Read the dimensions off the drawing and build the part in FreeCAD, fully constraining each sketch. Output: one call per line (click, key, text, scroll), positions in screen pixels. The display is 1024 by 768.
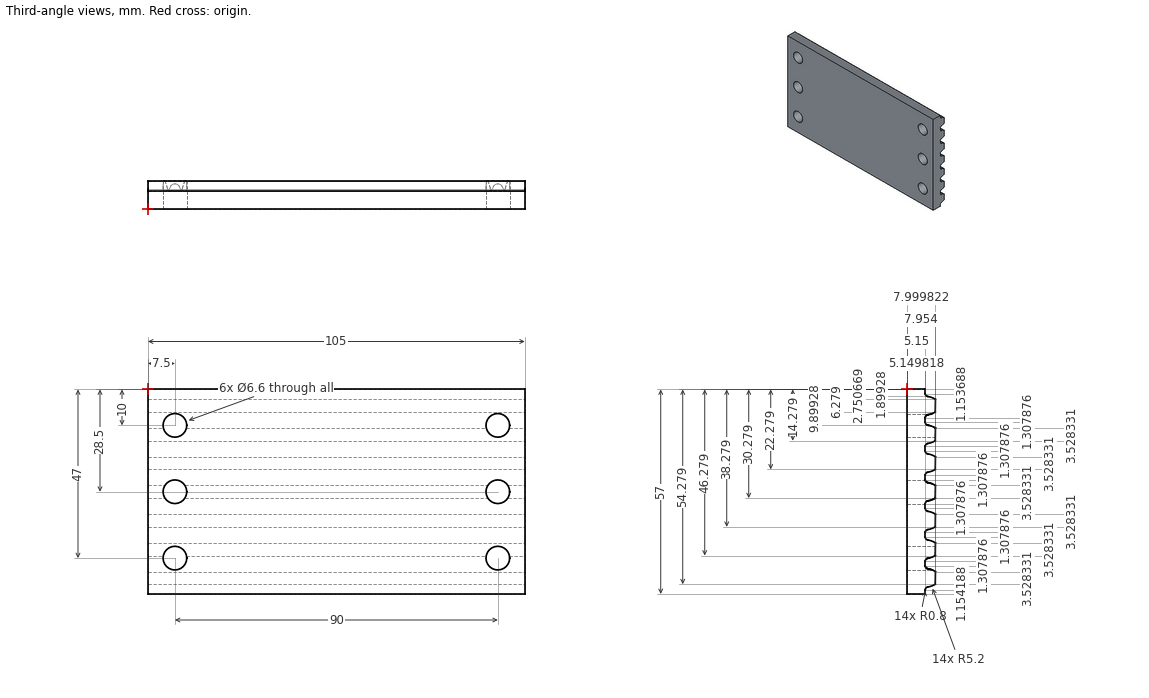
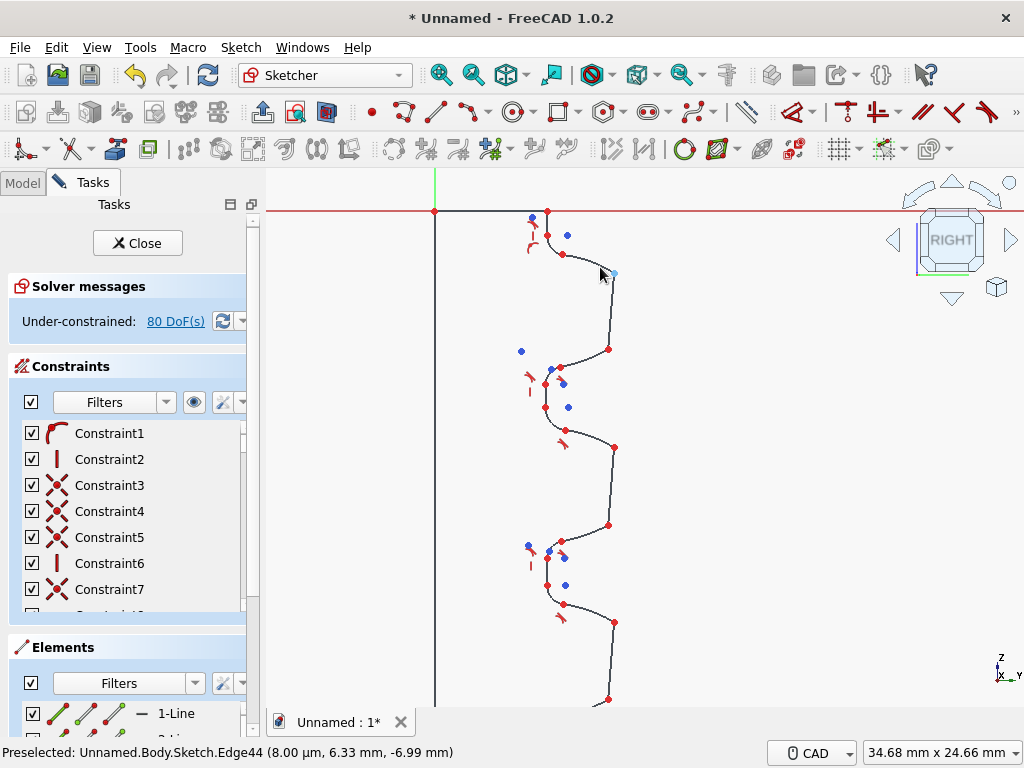
click(600, 265)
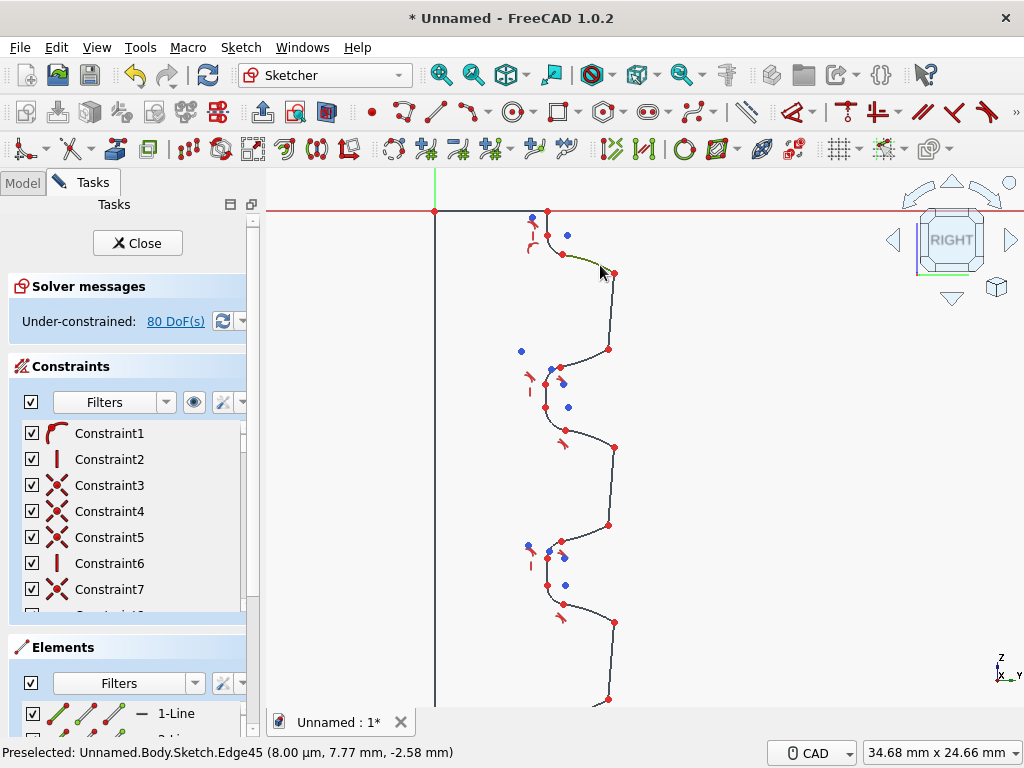
click(551, 248)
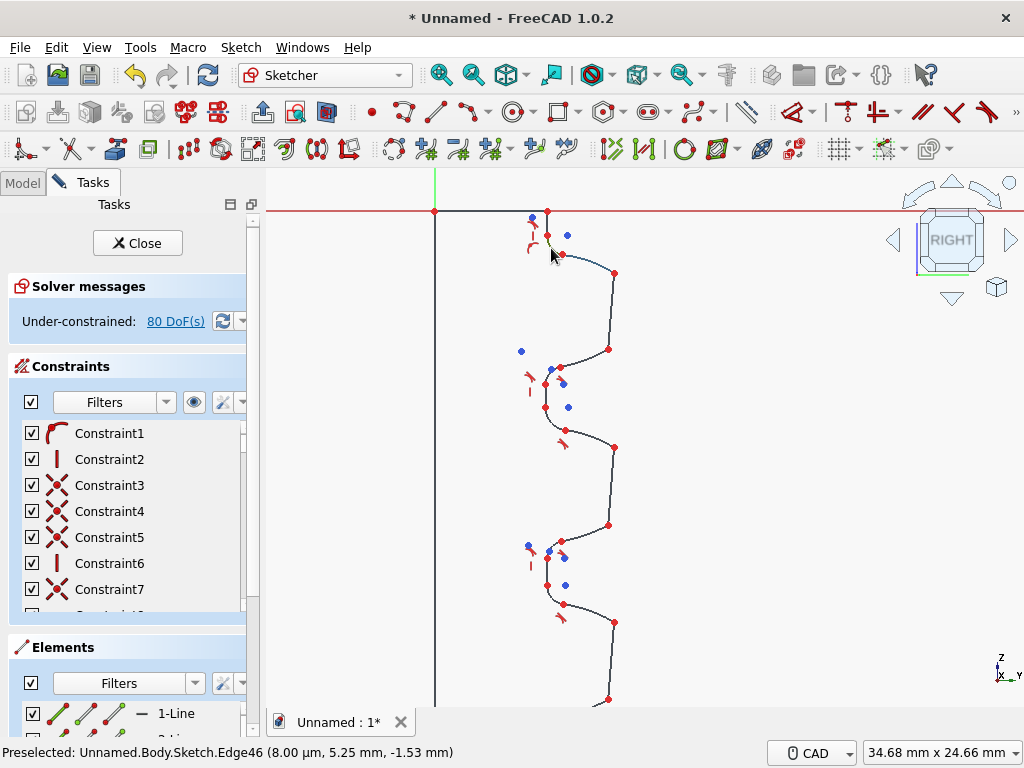
click(988, 112)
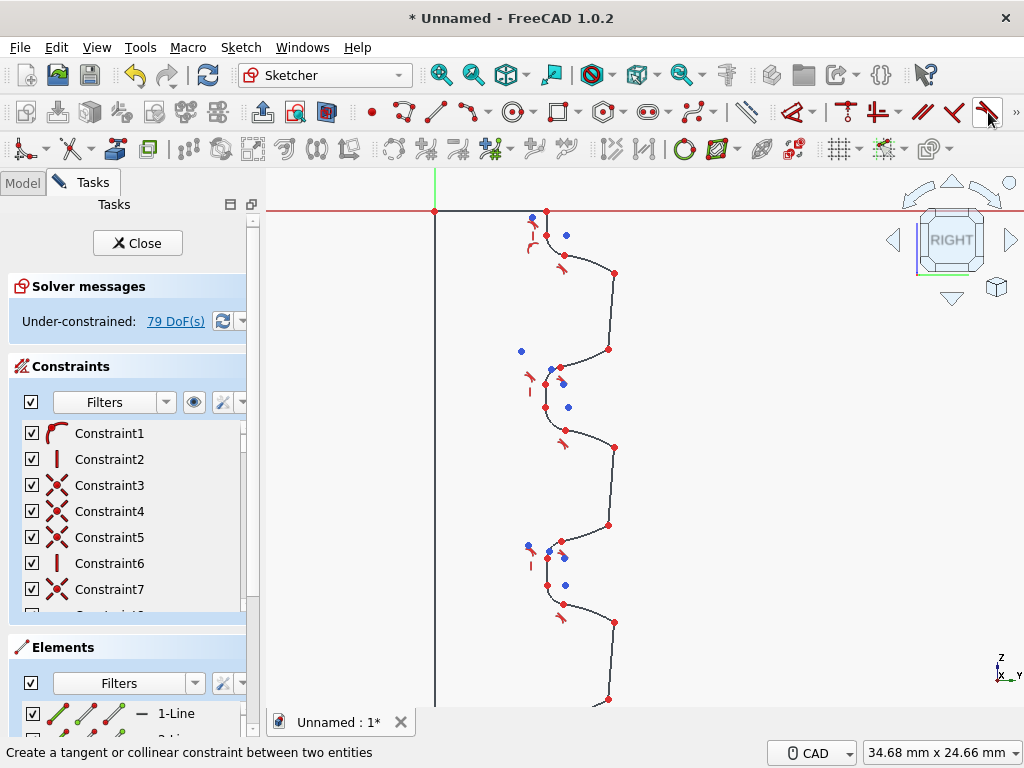
scroll(600, 267, down, 6)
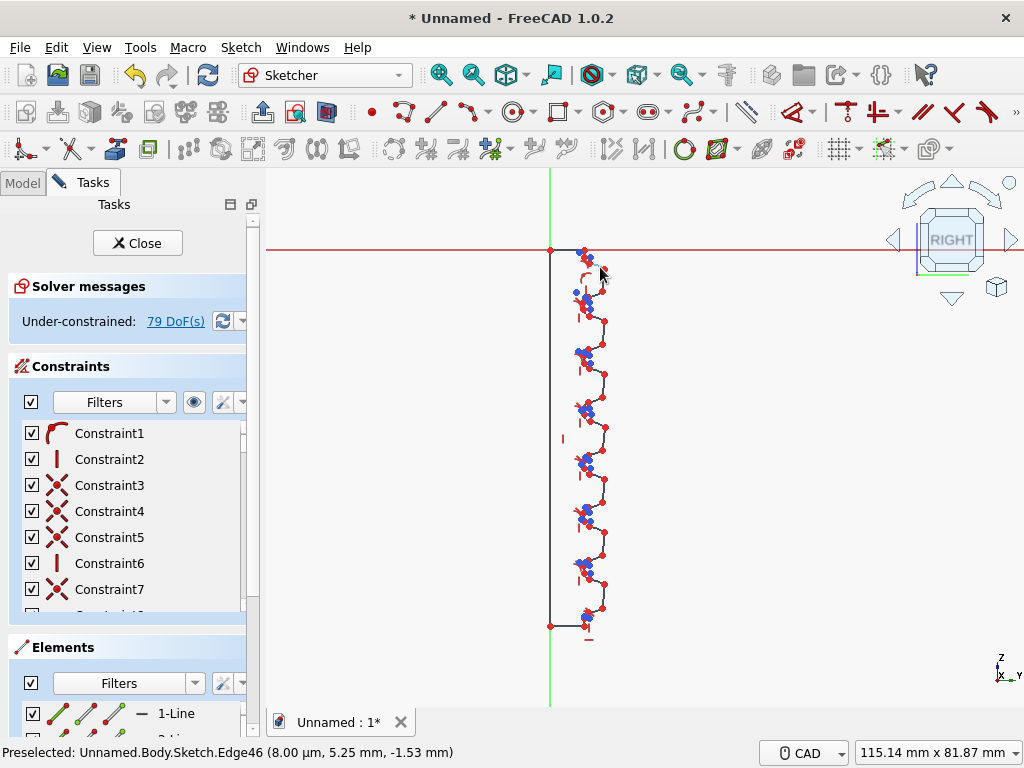
scroll(593, 612, up, 6)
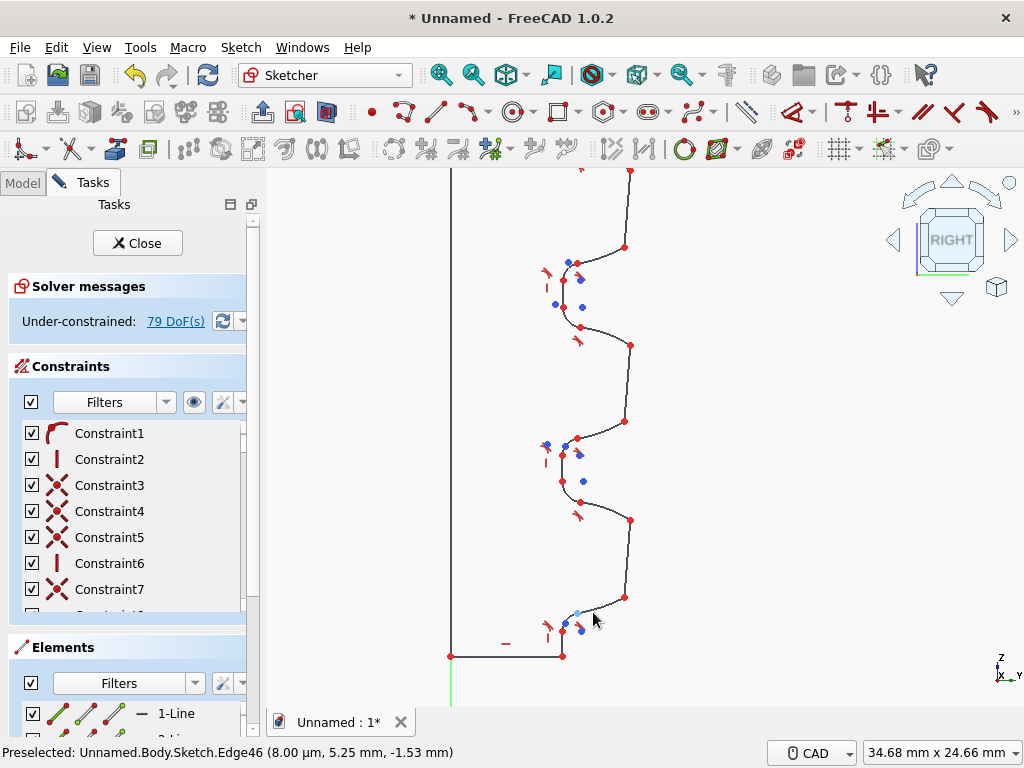
click(592, 610)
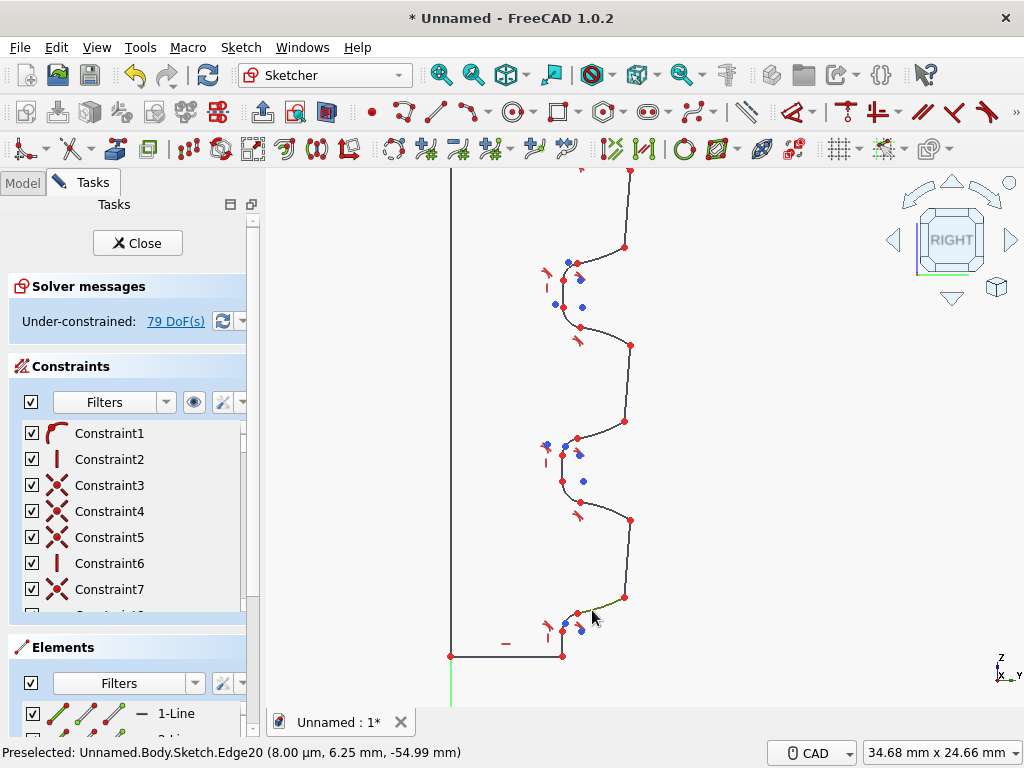
click(616, 512)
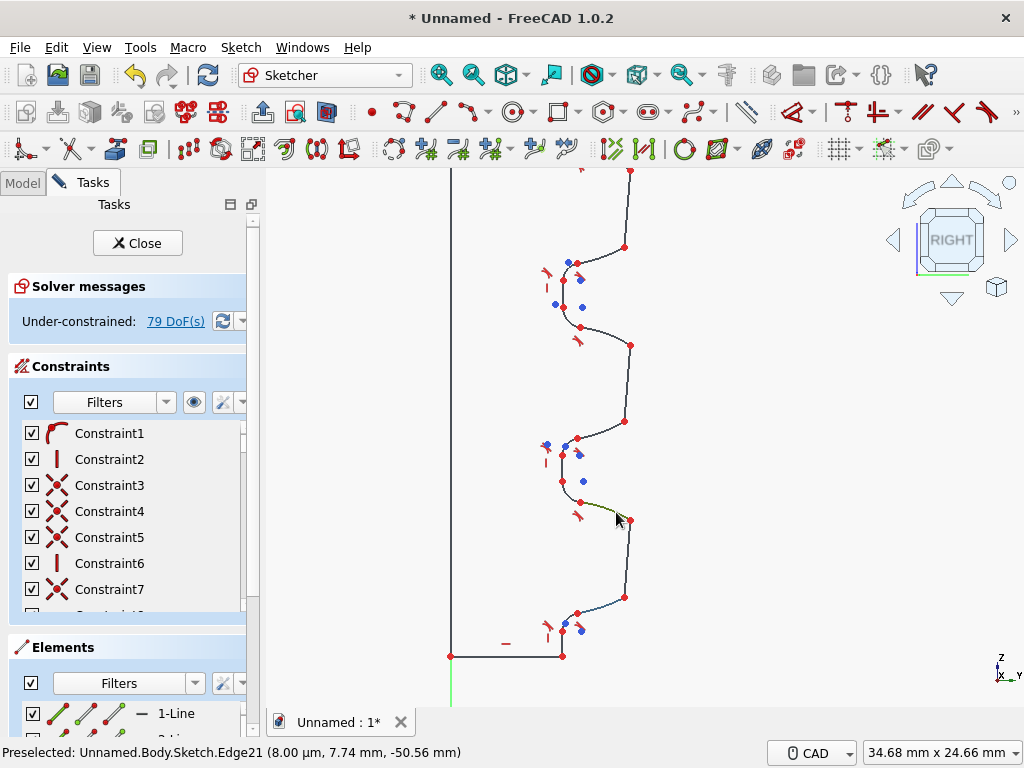
click(592, 435)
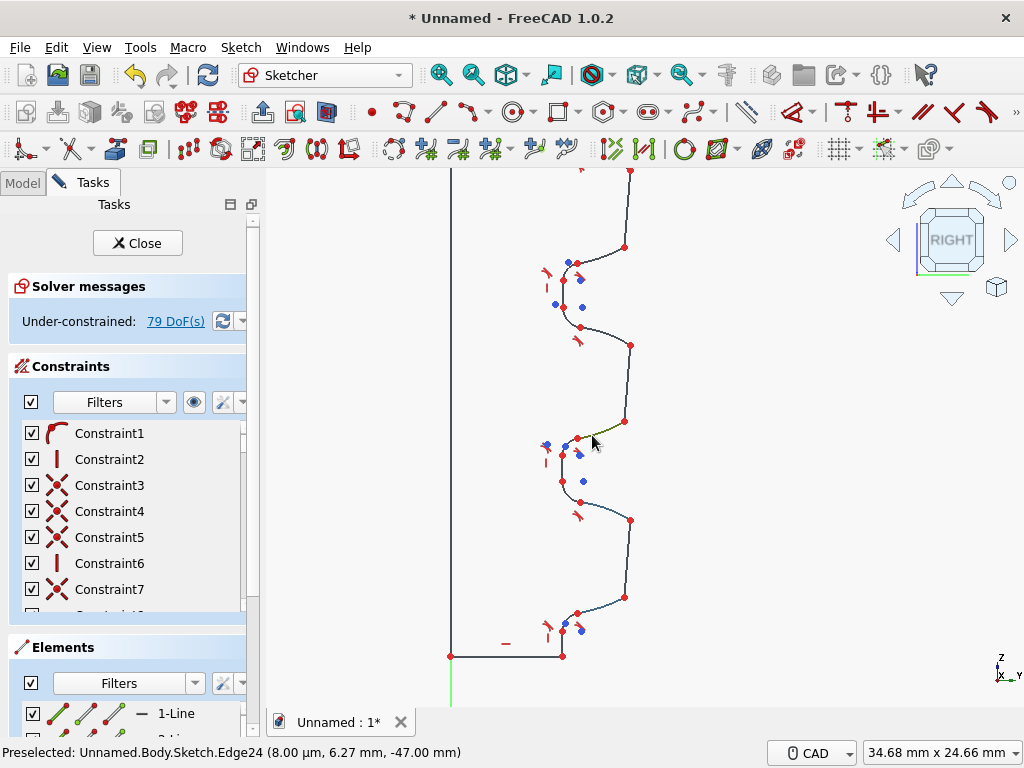
click(616, 338)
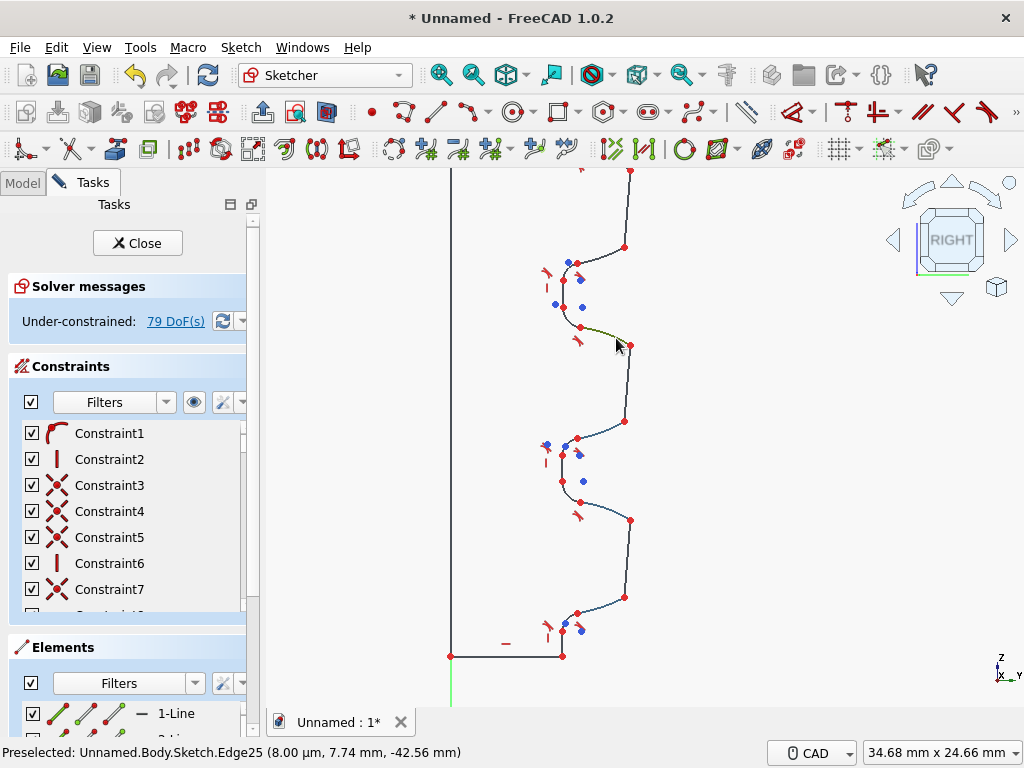
click(592, 260)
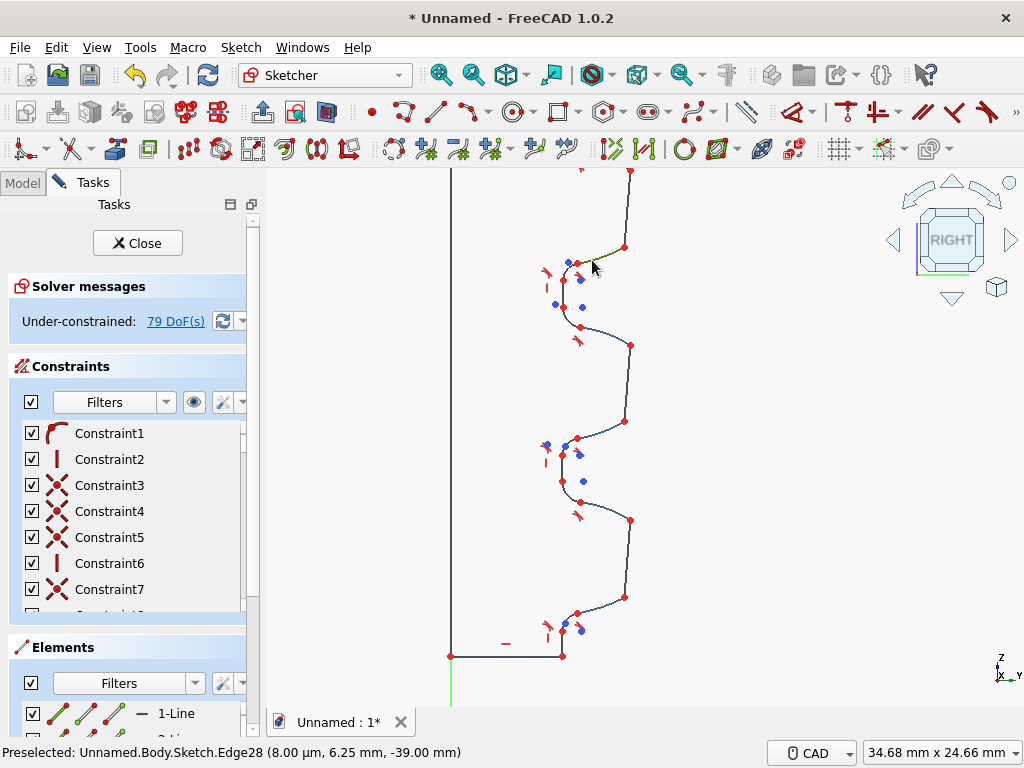
scroll(593, 612, down, 6)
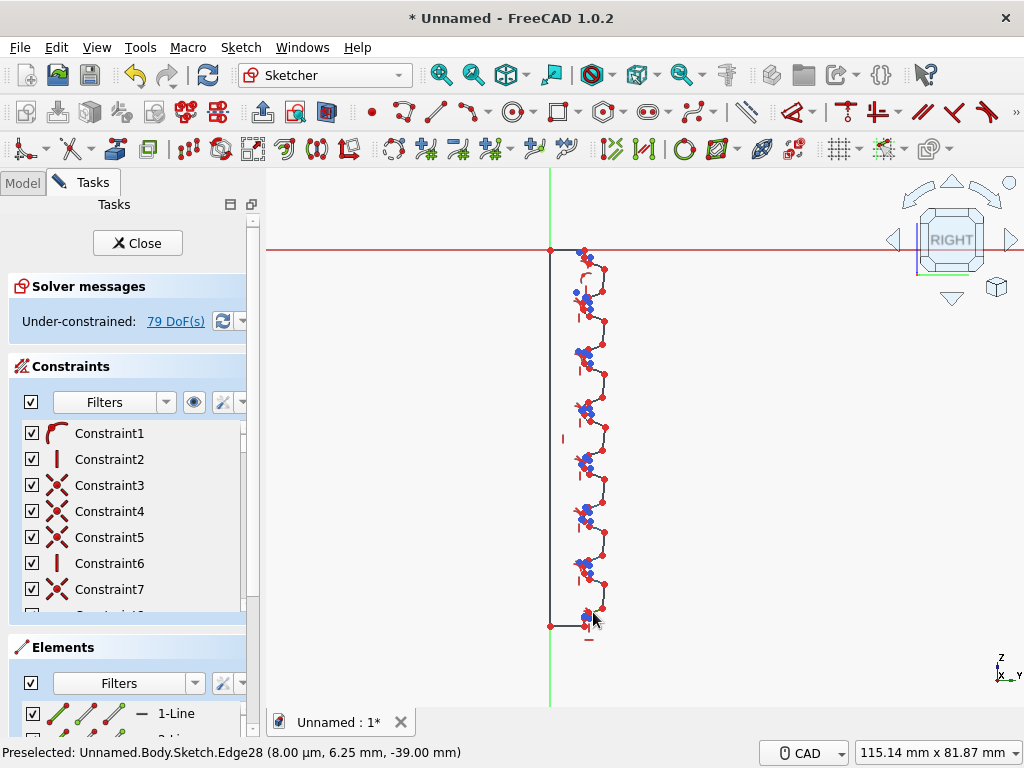
scroll(600, 477, up, 6)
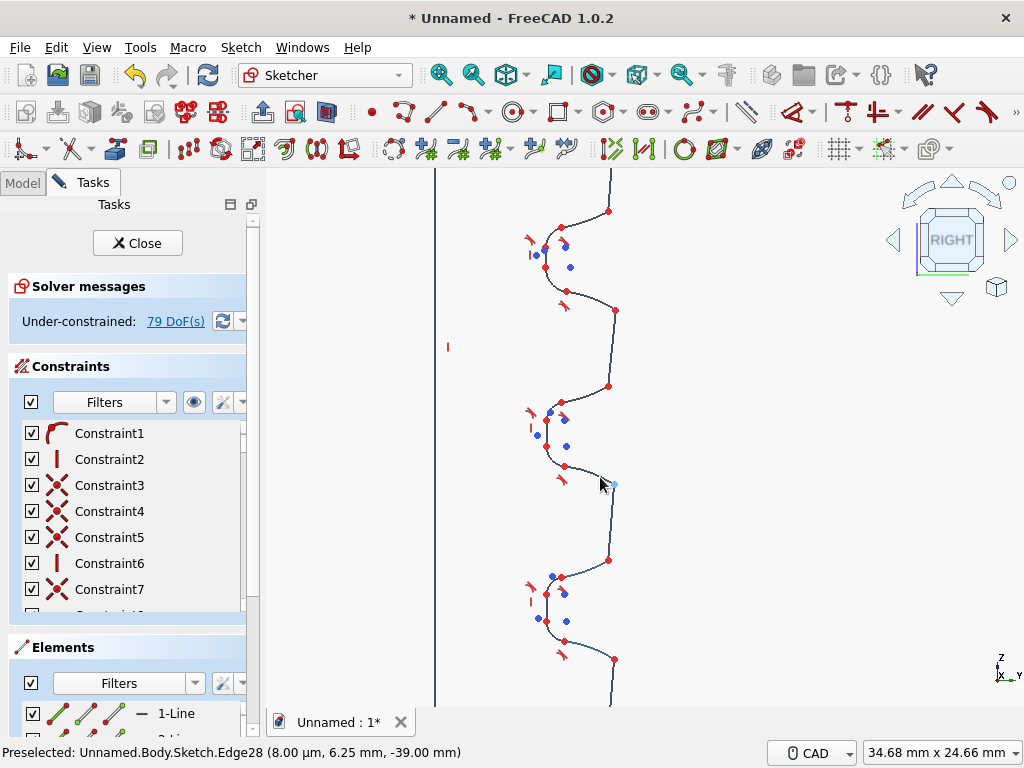
click(600, 477)